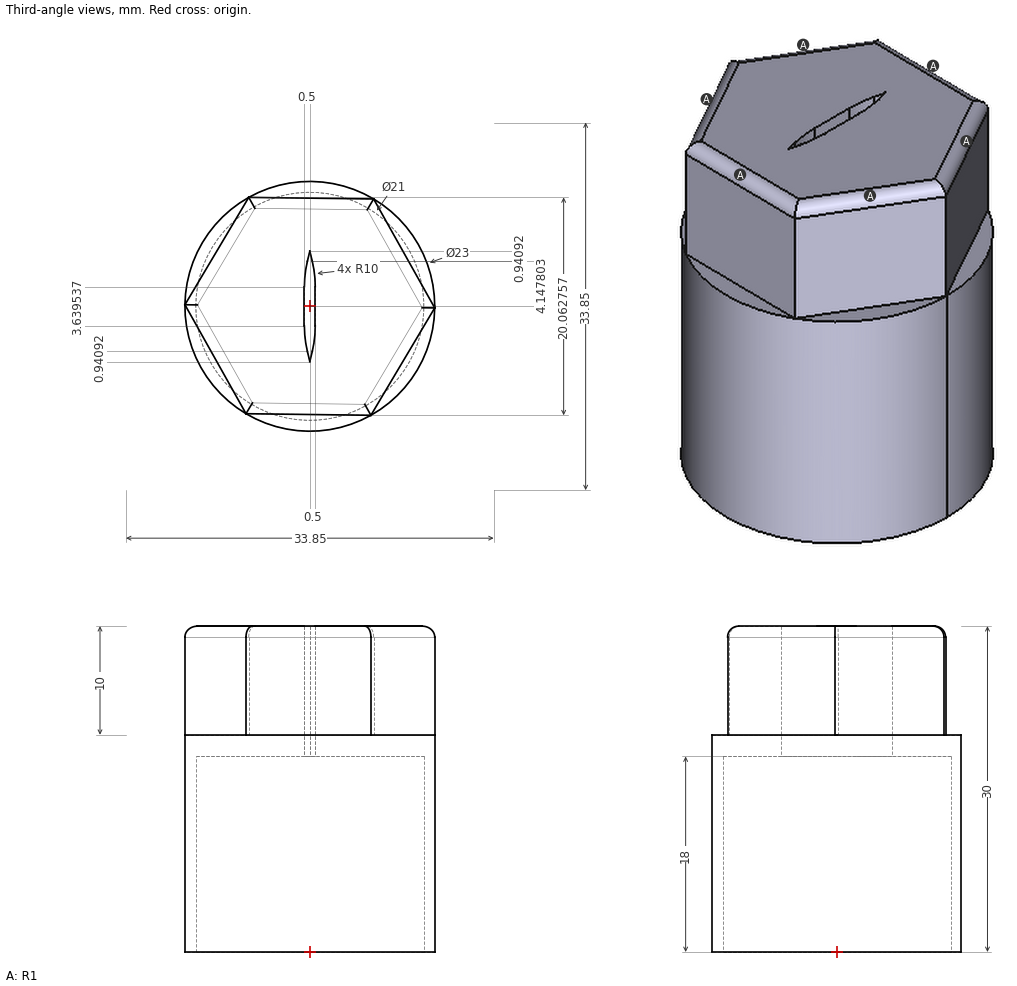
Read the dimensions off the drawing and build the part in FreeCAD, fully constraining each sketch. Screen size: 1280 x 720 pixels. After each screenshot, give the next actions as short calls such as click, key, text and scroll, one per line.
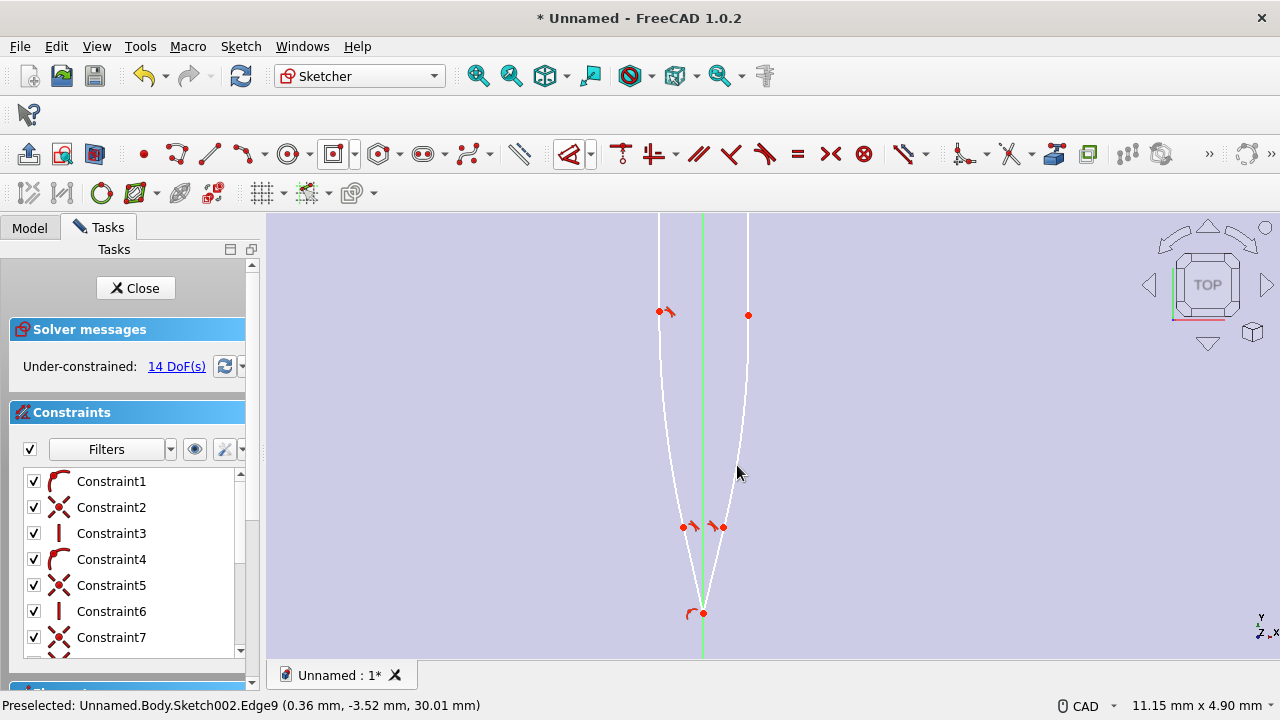
click(748, 250)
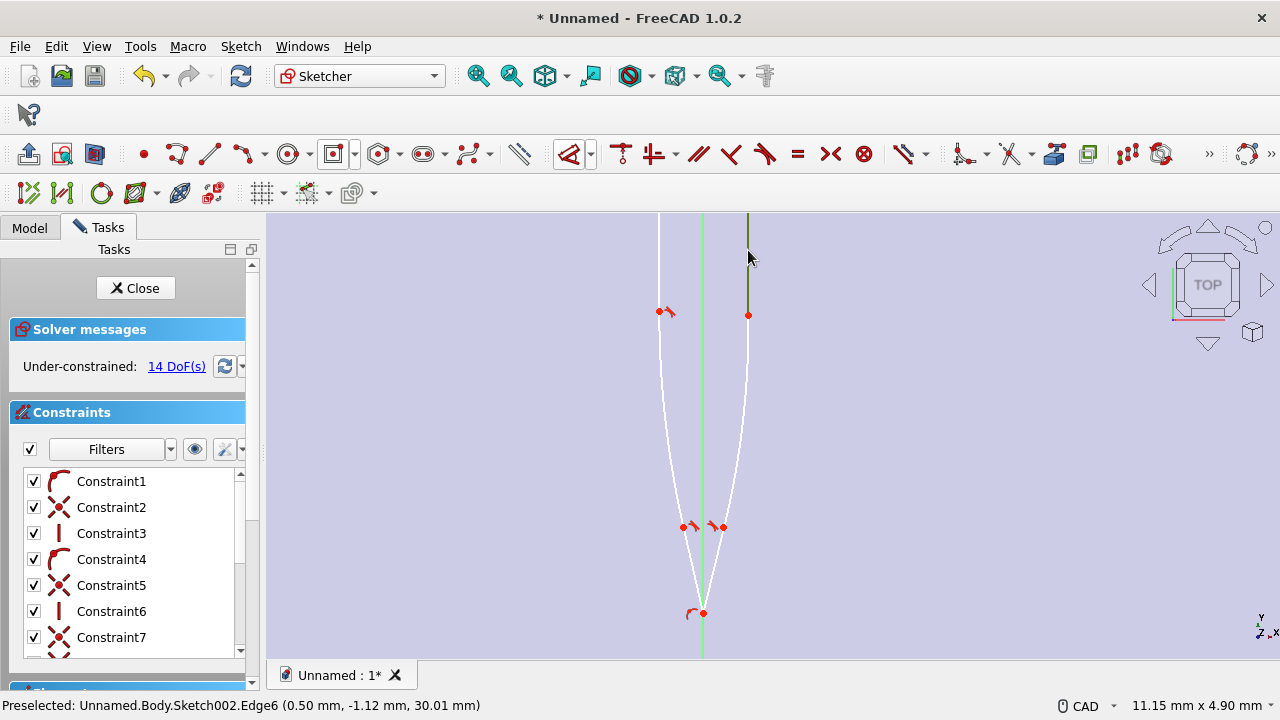
click(737, 465)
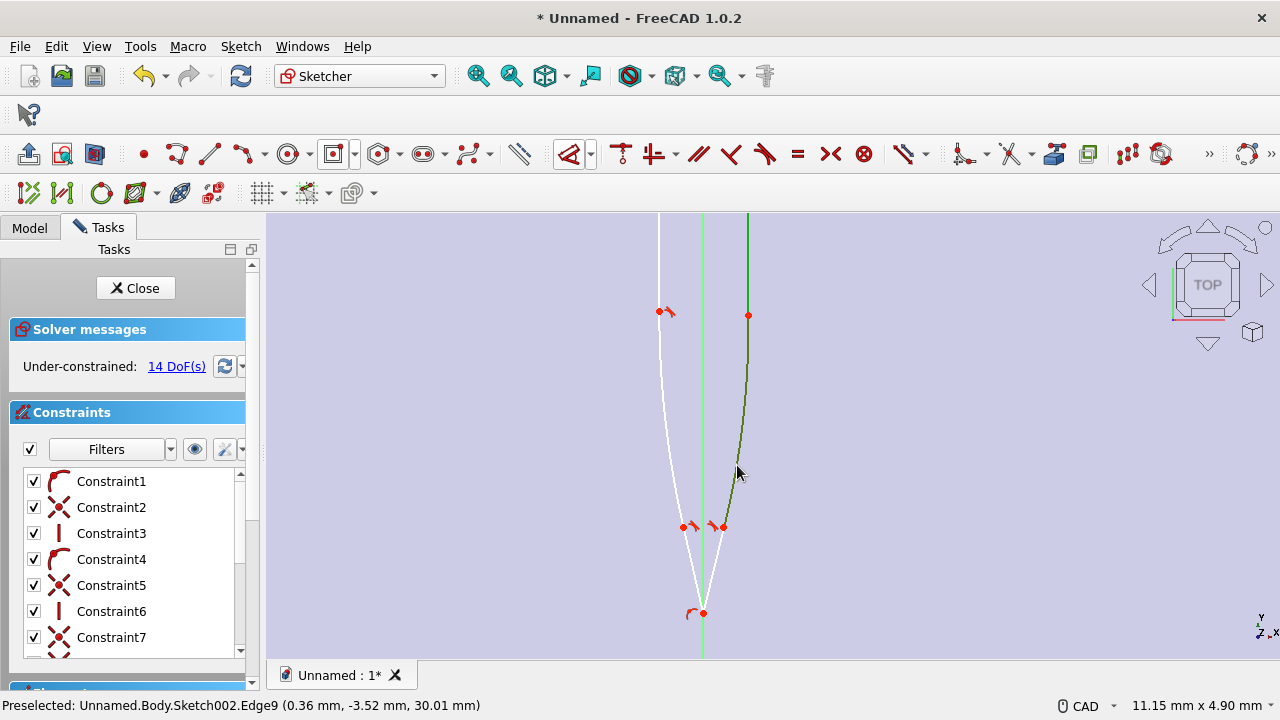
click(765, 154)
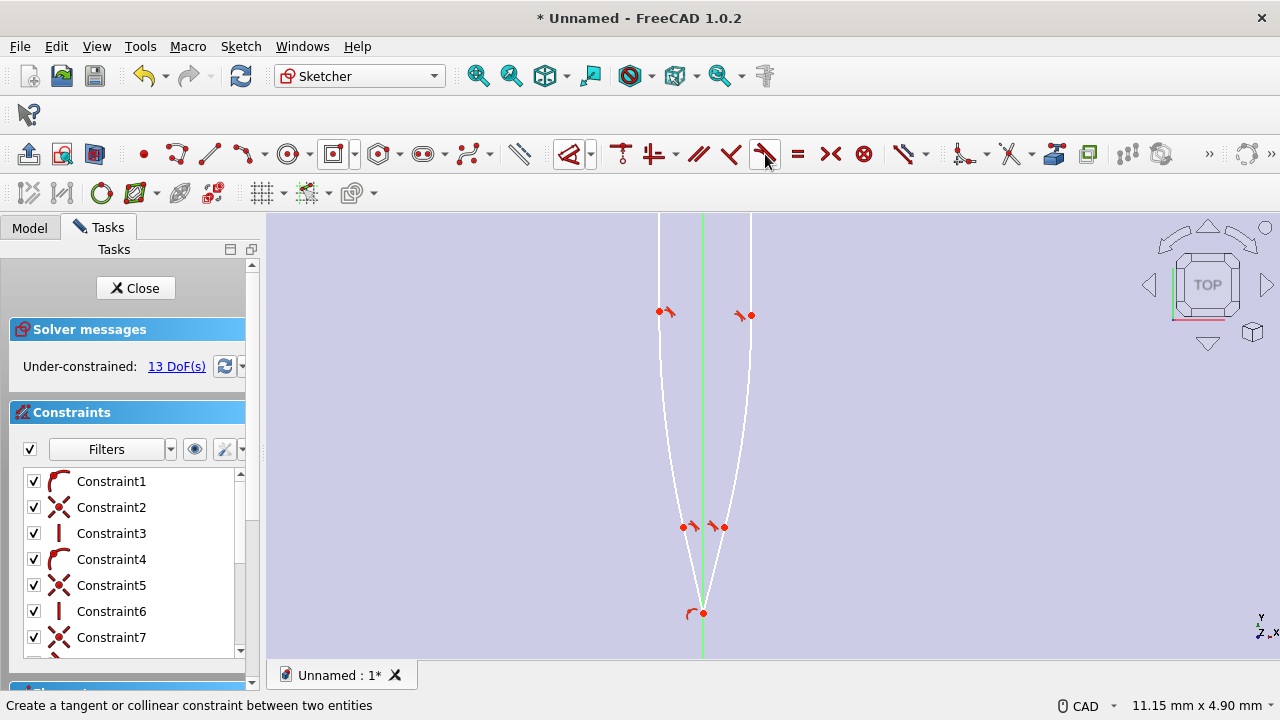
click(751, 250)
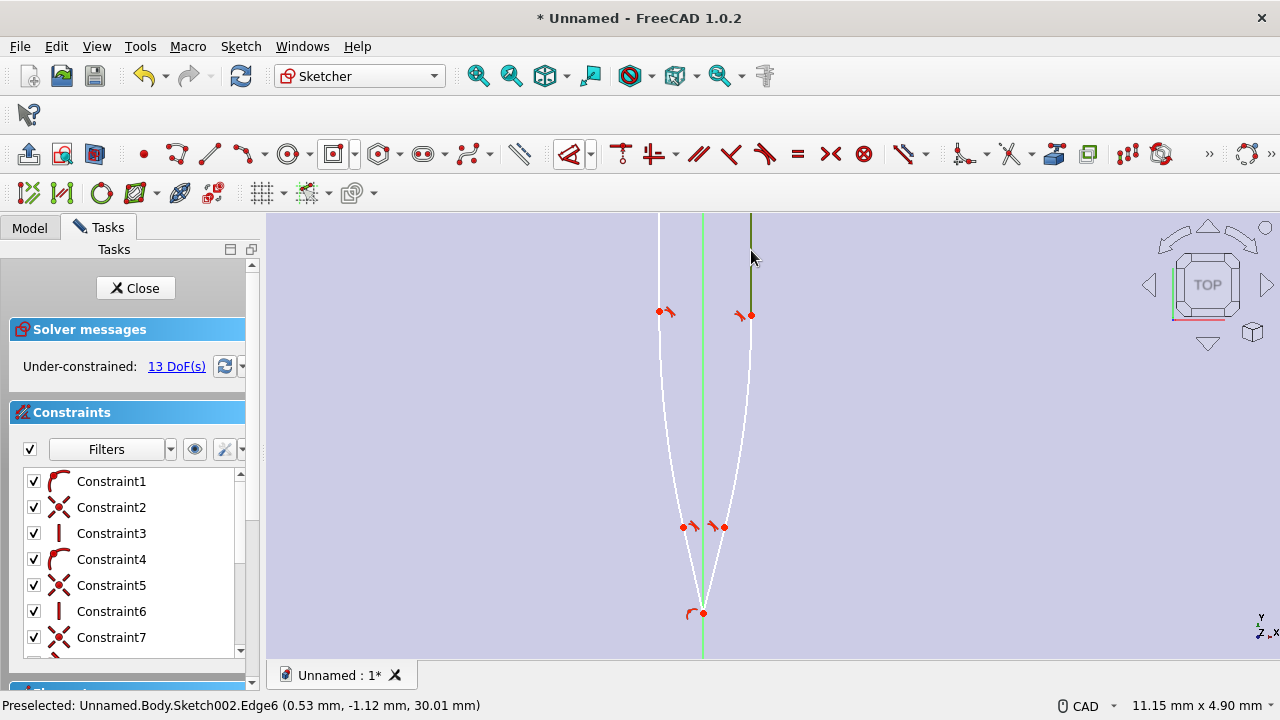
scroll(705, 560, down, 6)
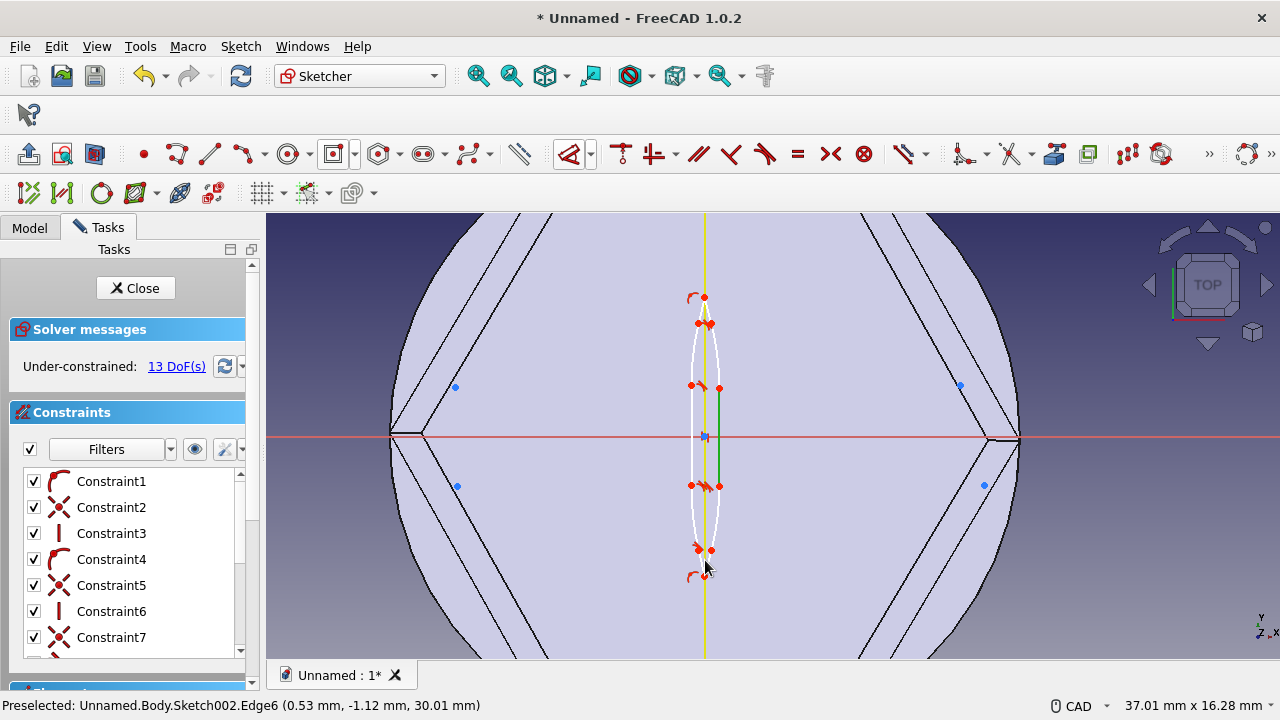
click(719, 369)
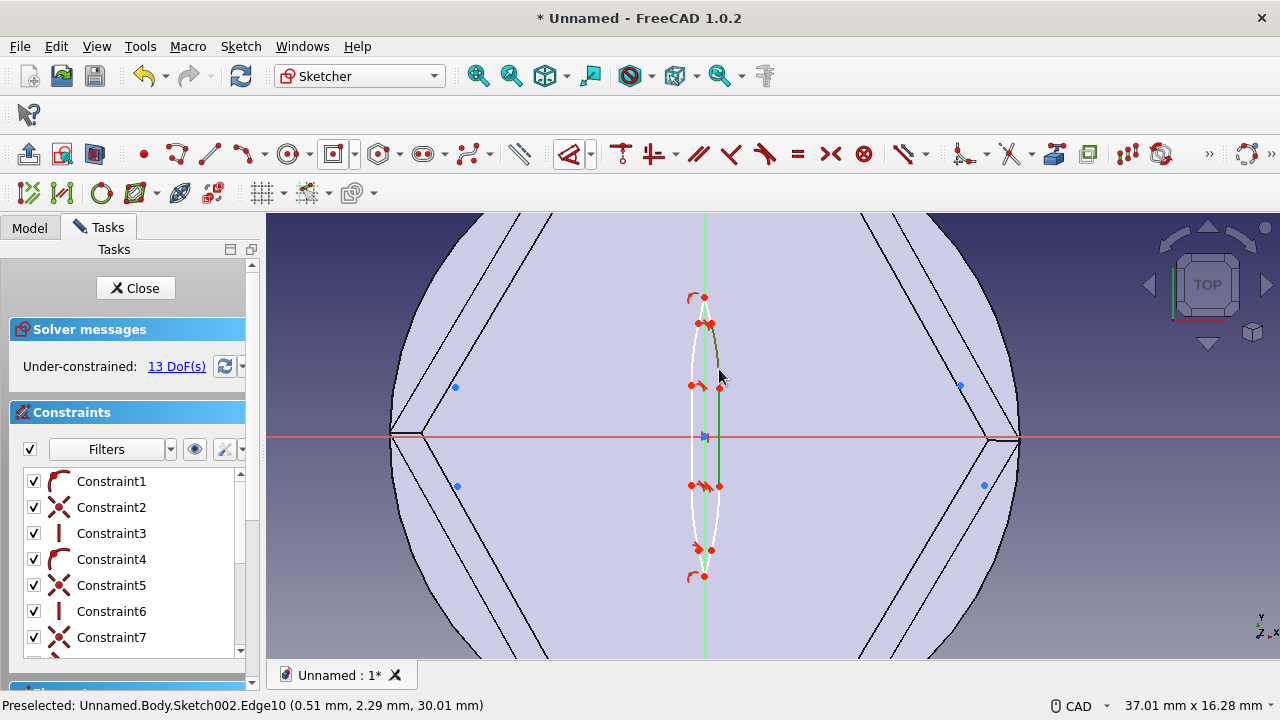
click(765, 154)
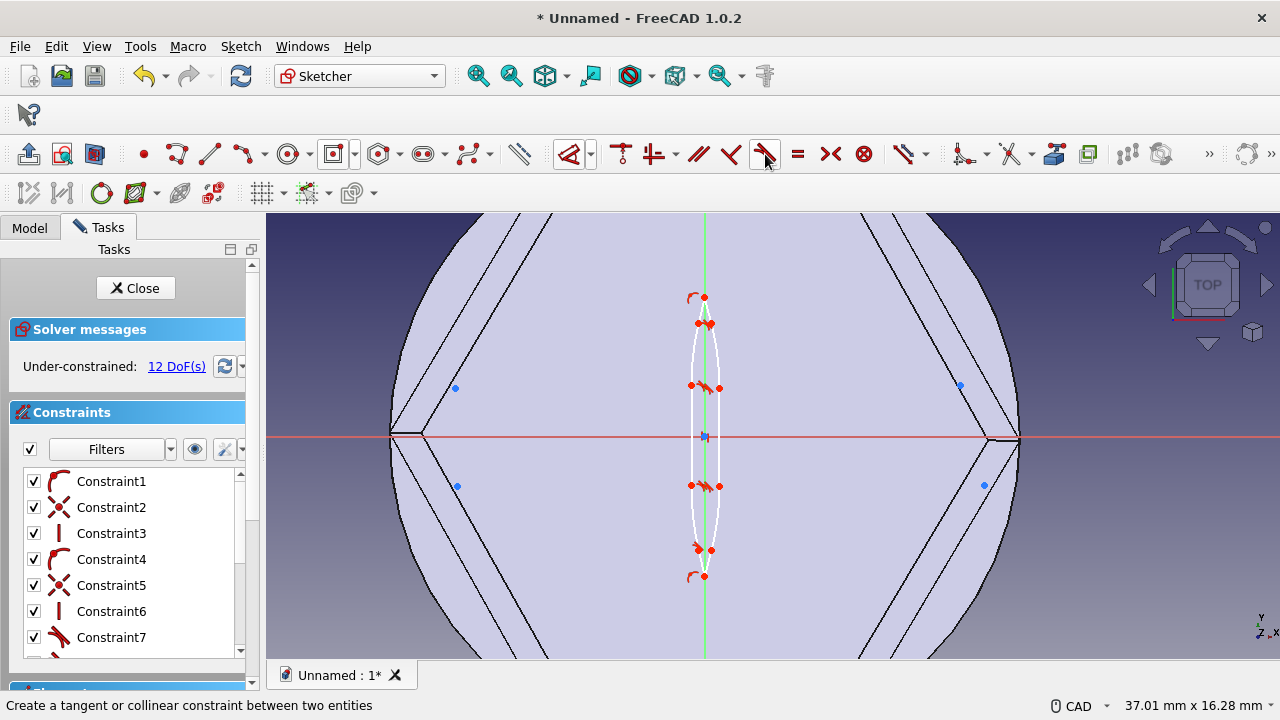
scroll(695, 342, up, 2)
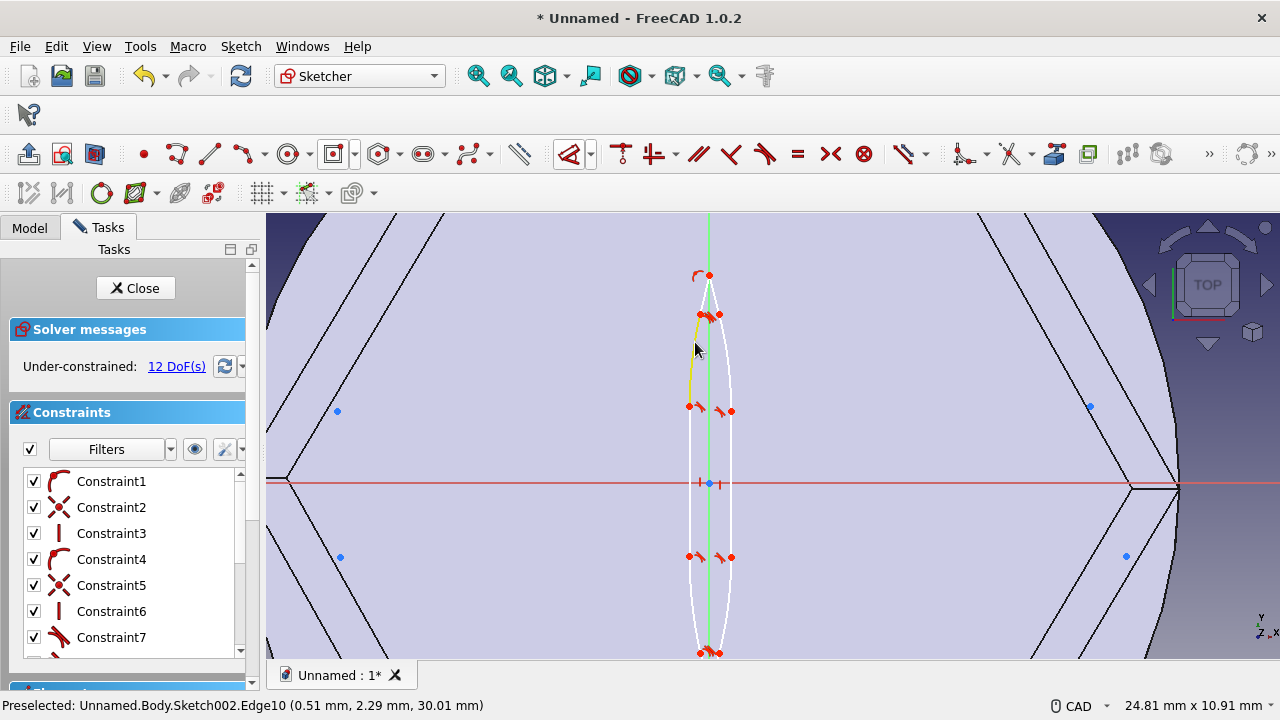
click(695, 342)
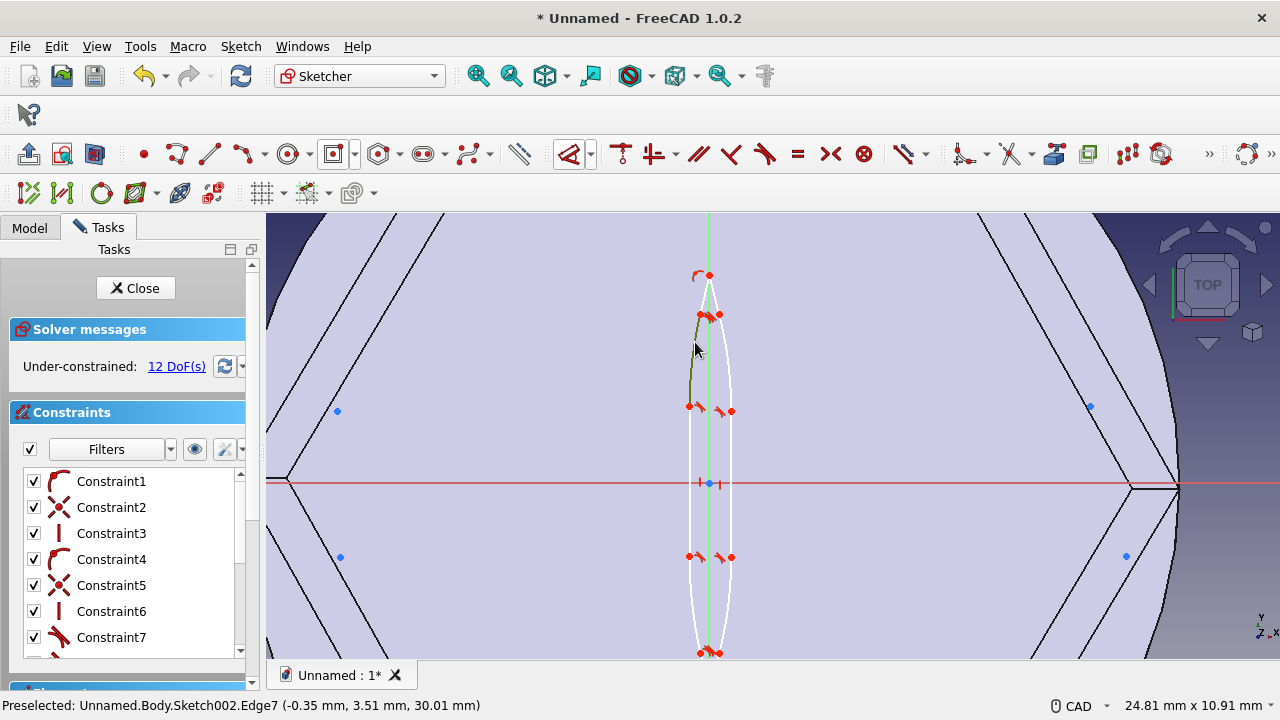
click(691, 586)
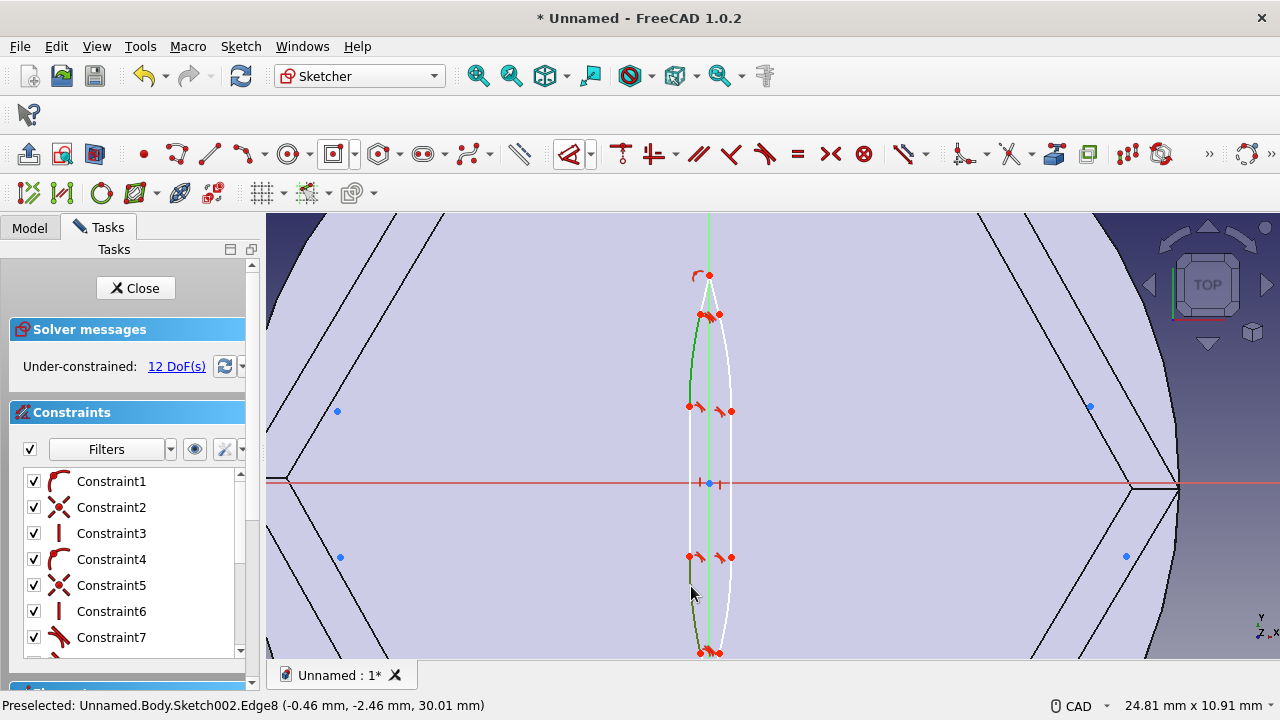
click(725, 625)